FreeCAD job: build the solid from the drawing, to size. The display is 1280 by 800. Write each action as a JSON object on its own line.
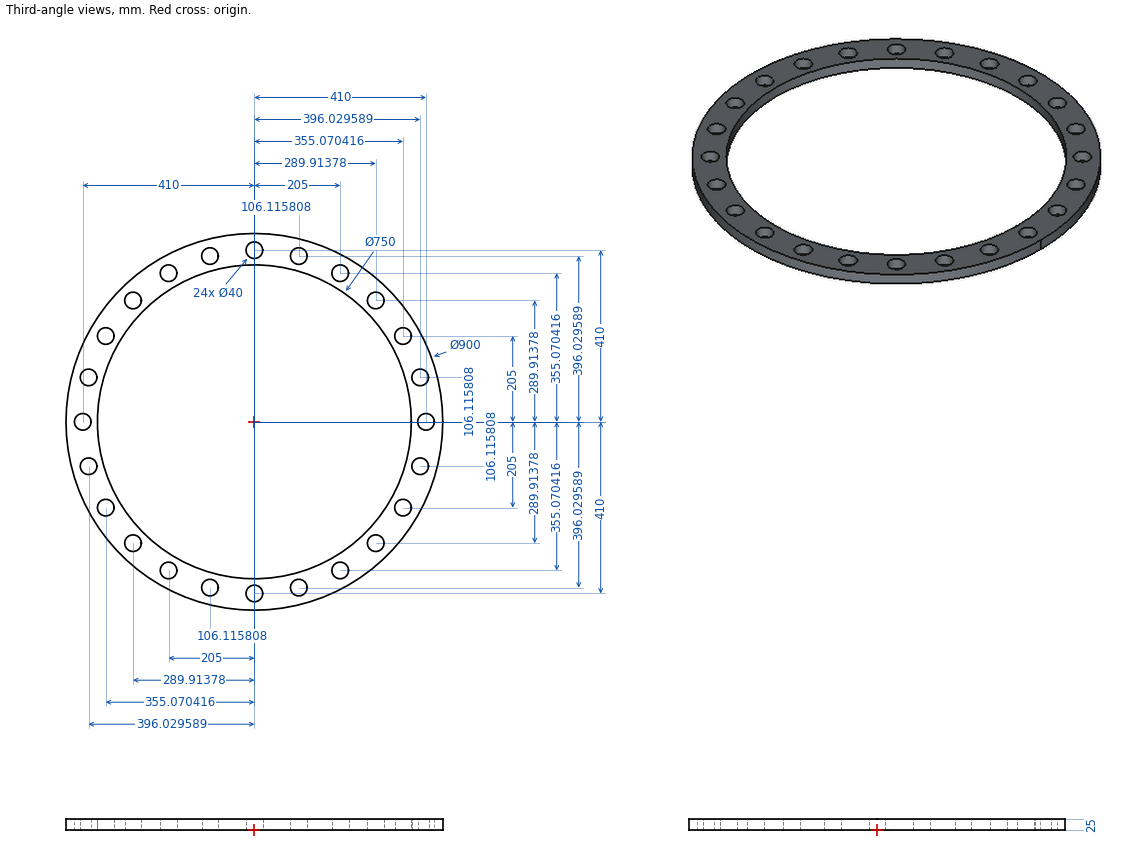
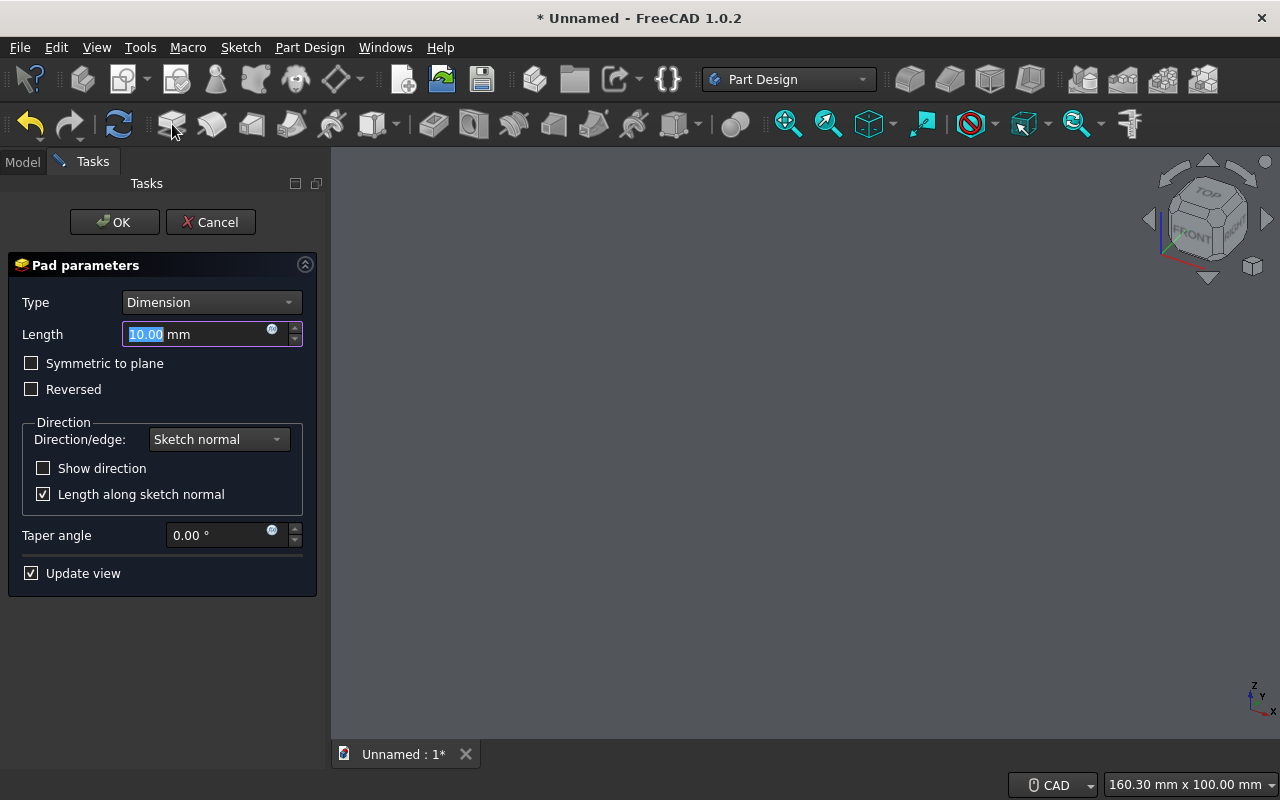
{"action": "type", "text": "25"}
{"action": "key", "text": "Tab"}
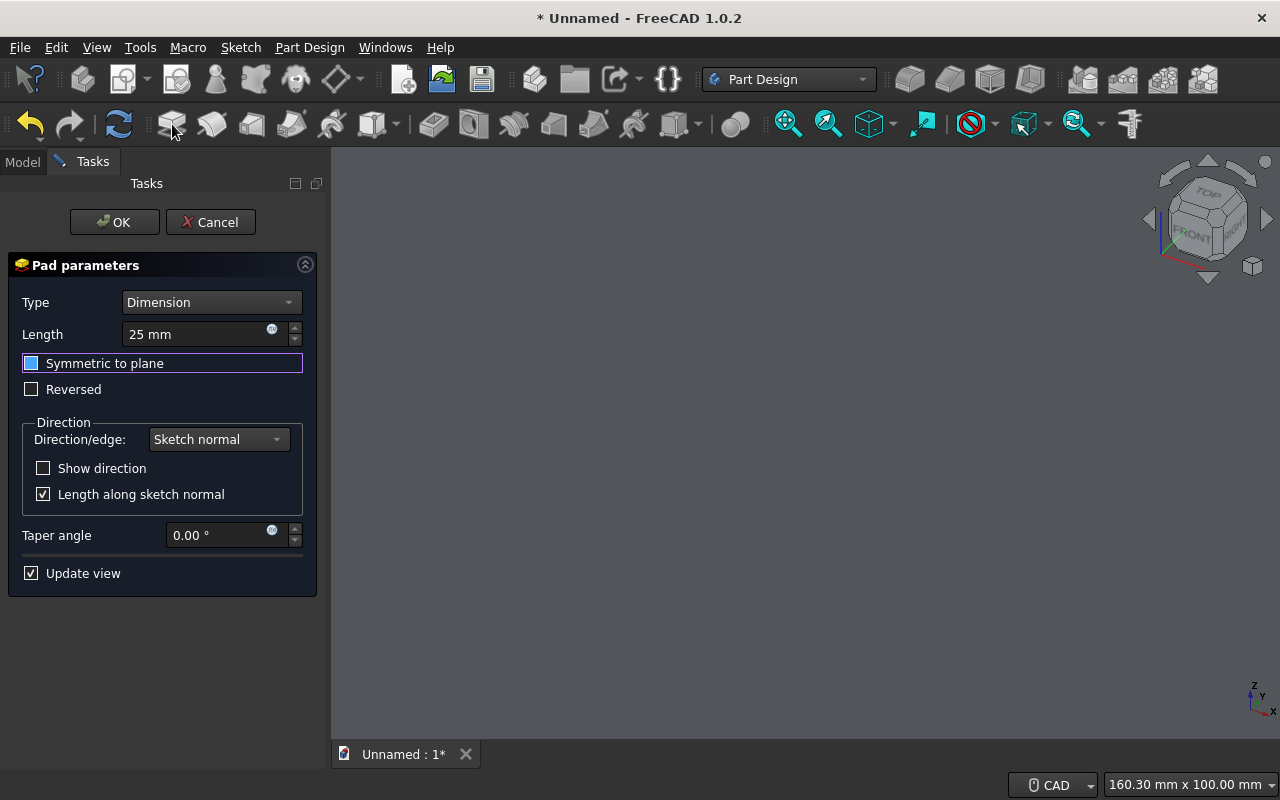
{"action": "left_click", "coordinate": [115, 222]}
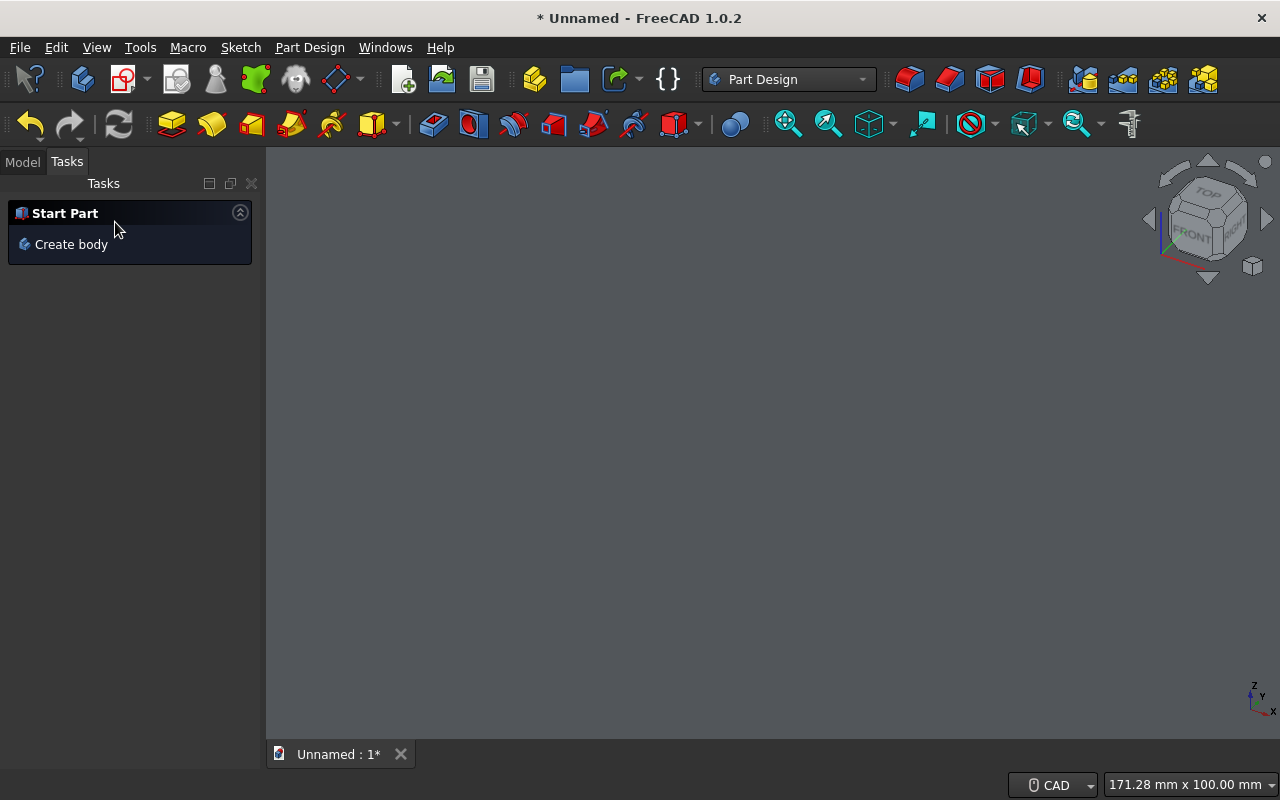
{"action": "left_click", "coordinate": [790, 124]}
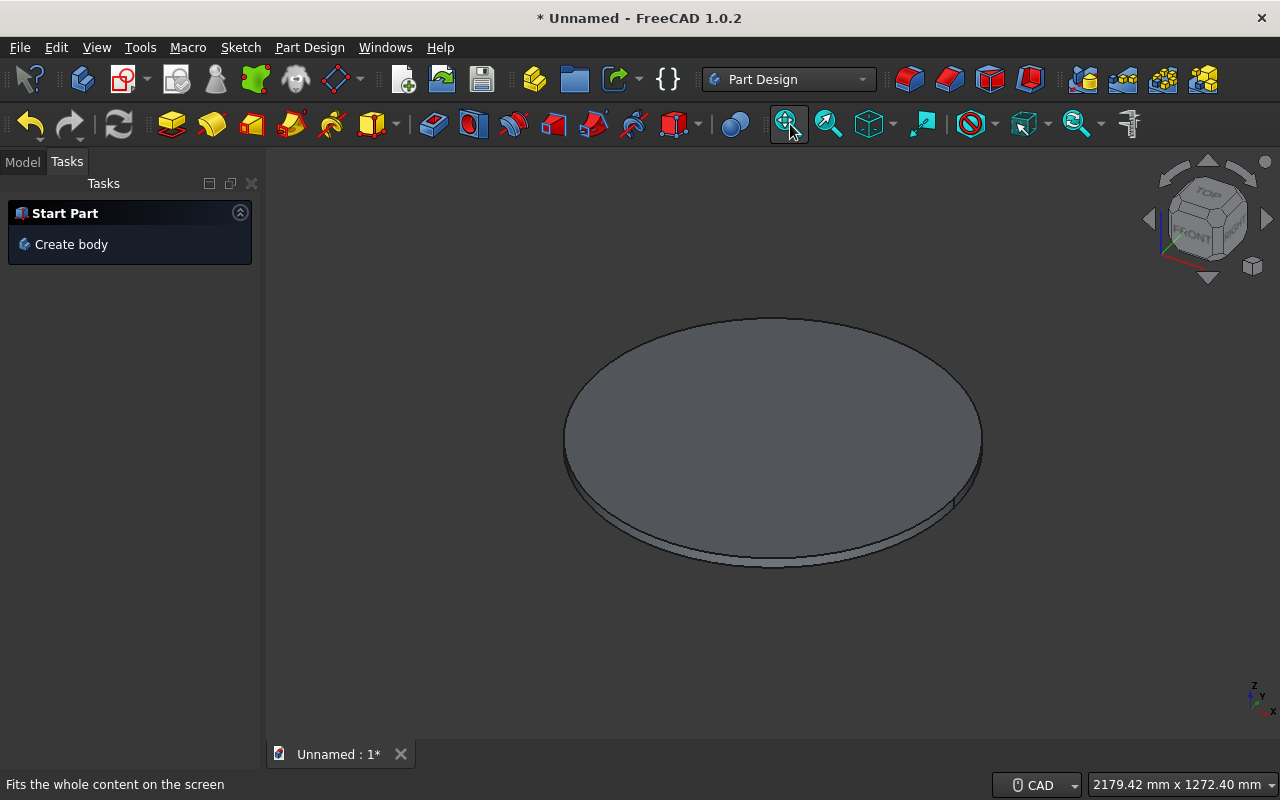
{"action": "left_click", "coordinate": [773, 437]}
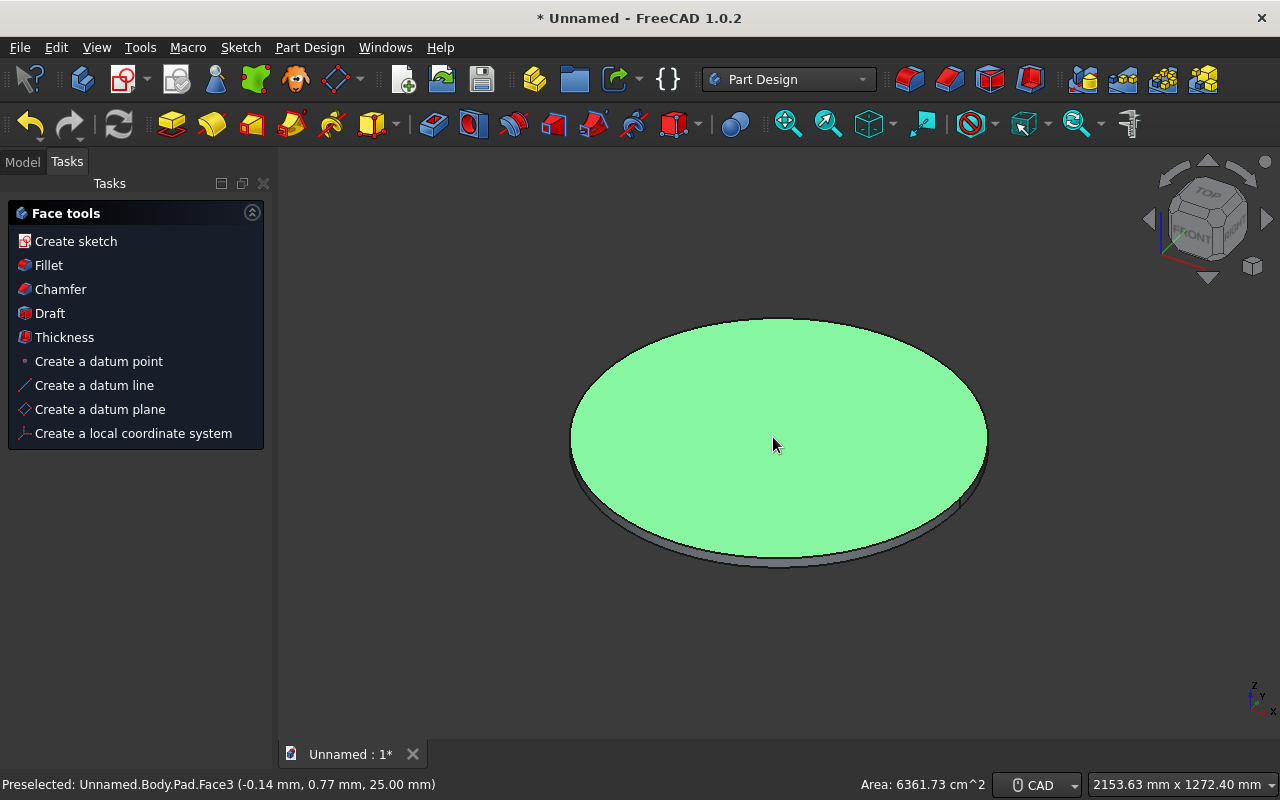
{"action": "left_click", "coordinate": [124, 80]}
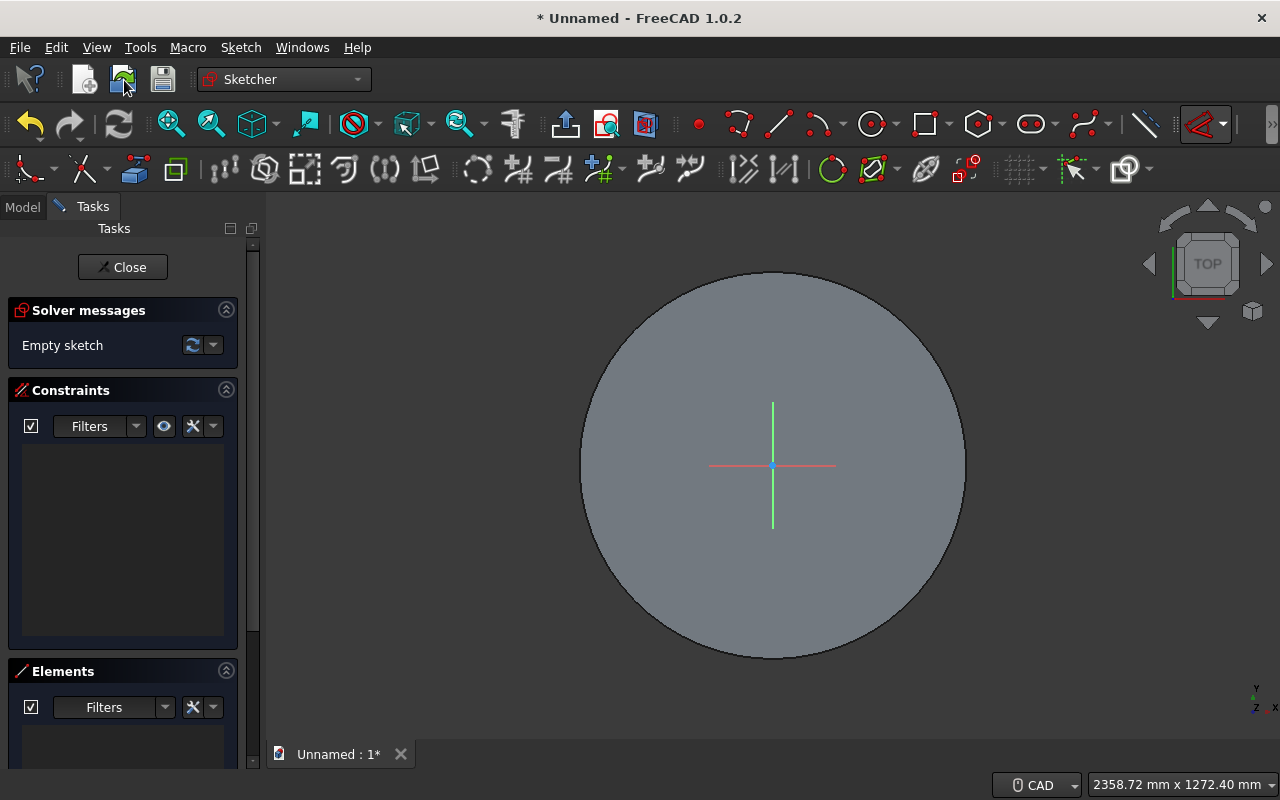
{"action": "left_click", "coordinate": [872, 124]}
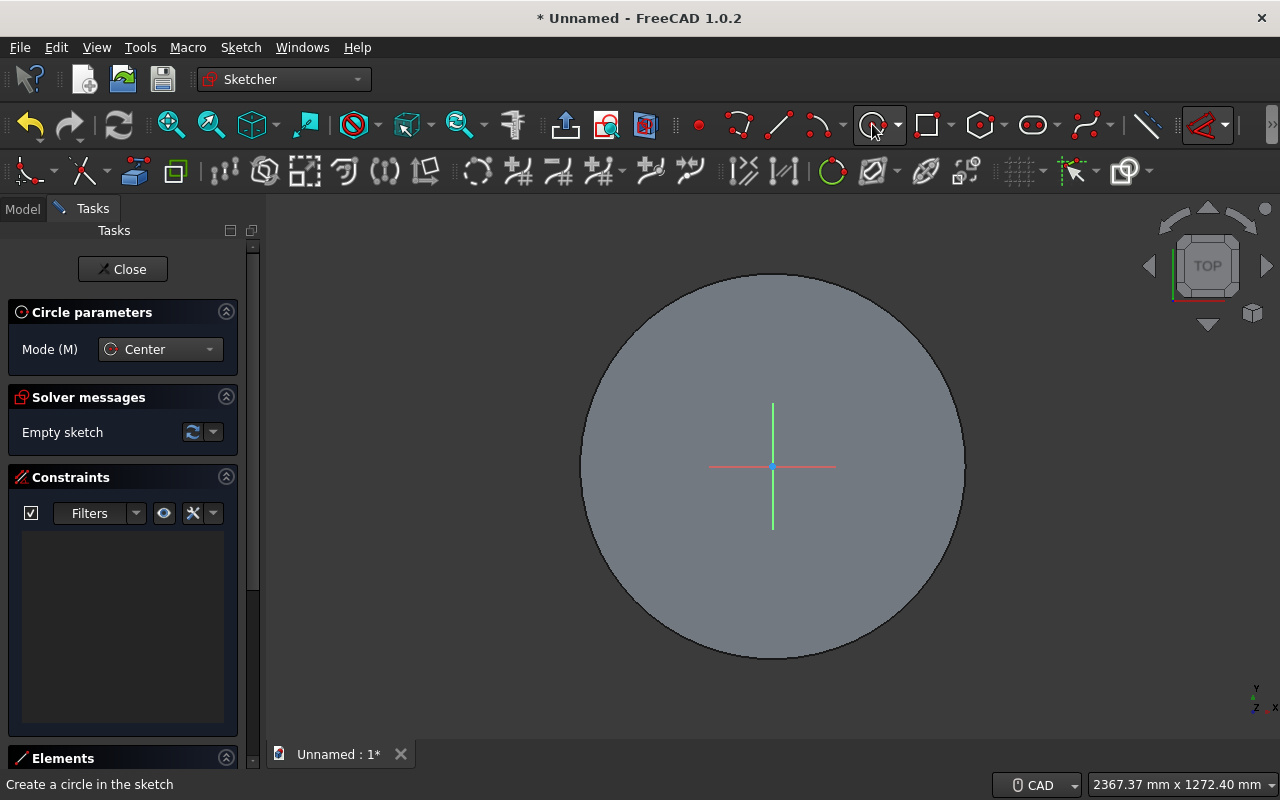
{"action": "scroll", "coordinate": [773, 291], "scroll_direction": "up", "scroll_amount": 5}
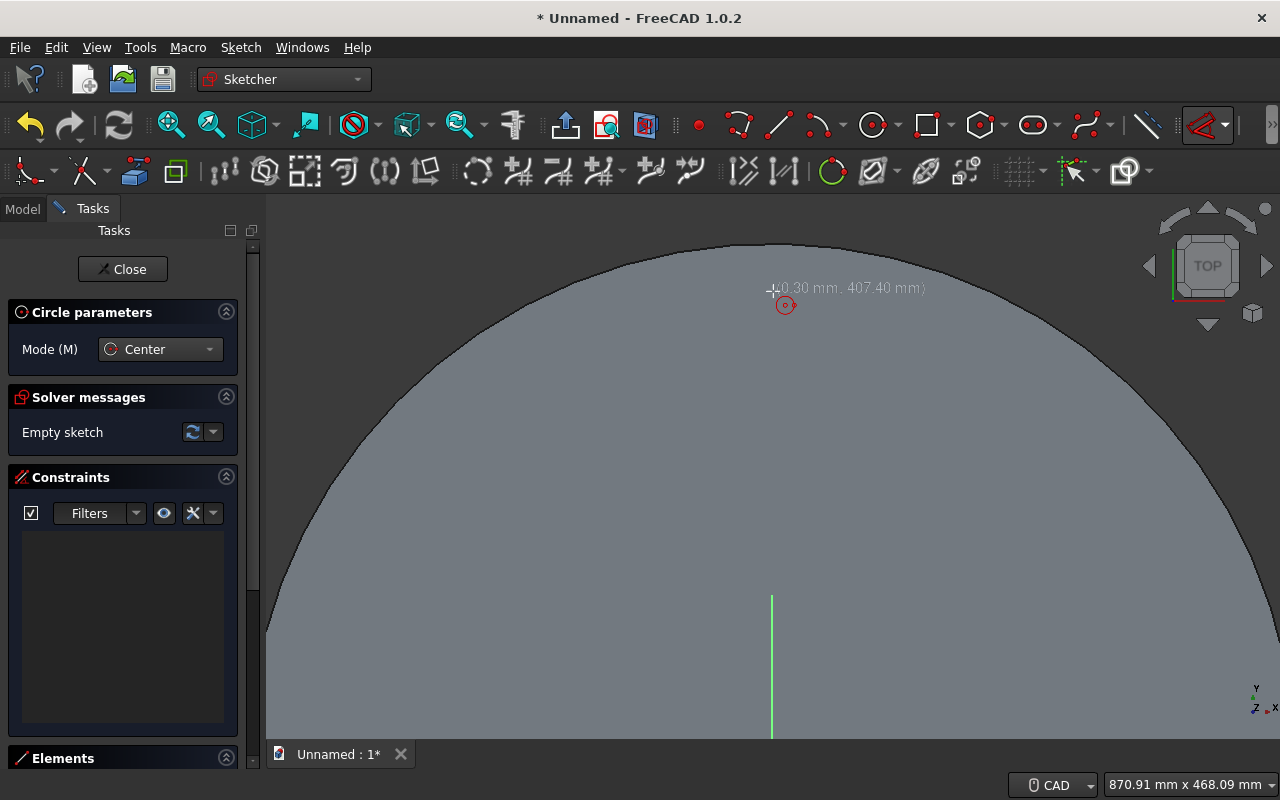
{"action": "left_click", "coordinate": [772, 290]}
{"action": "mouse_move", "coordinate": [788, 274]}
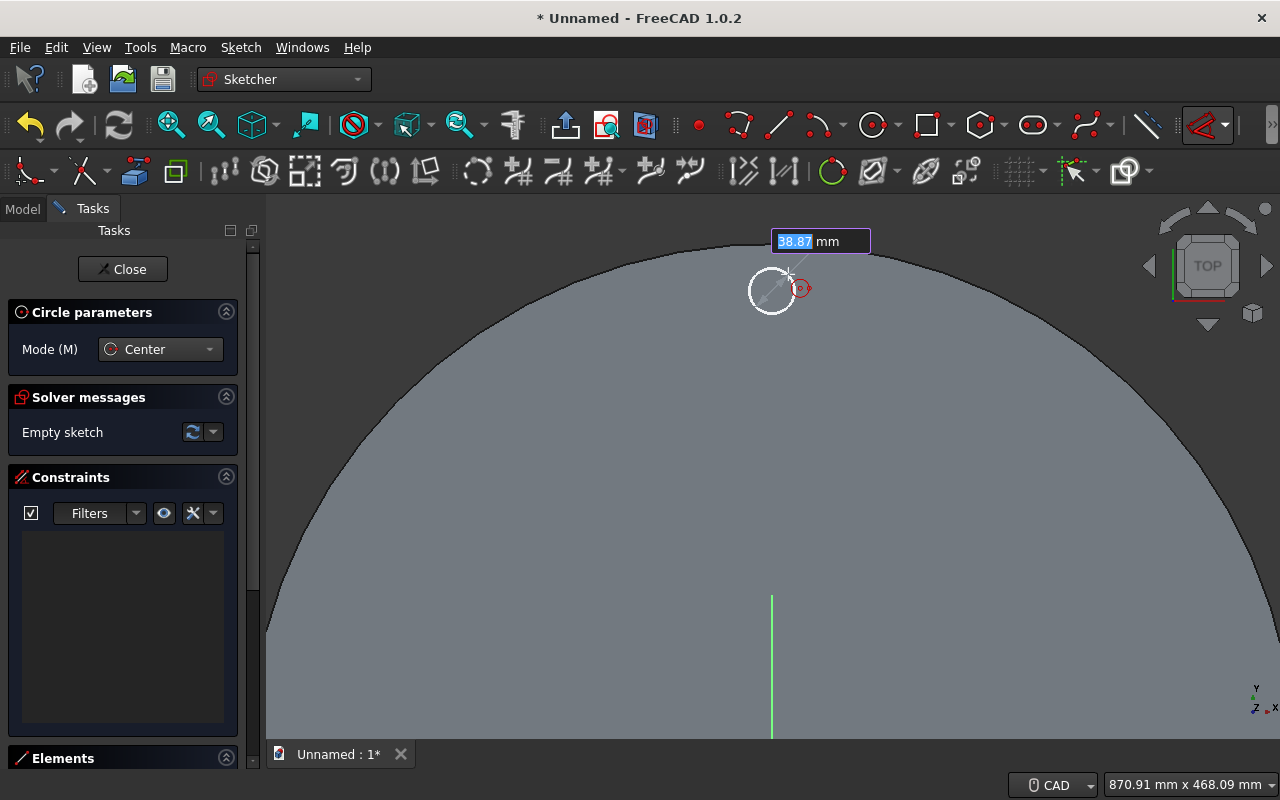
{"action": "type", "text": "40"}
{"action": "key", "text": "Return"}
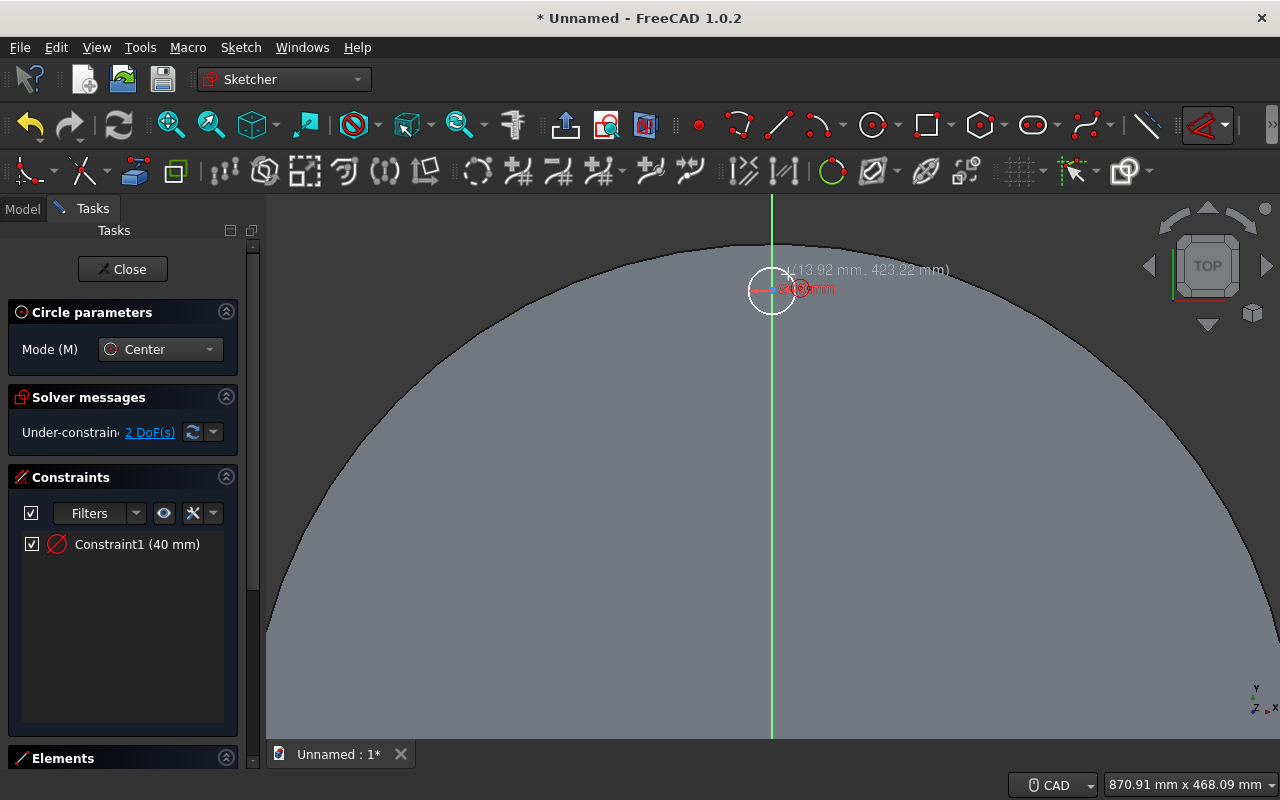
{"action": "left_click", "coordinate": [895, 307]}
{"action": "mouse_move", "coordinate": [912, 290]}